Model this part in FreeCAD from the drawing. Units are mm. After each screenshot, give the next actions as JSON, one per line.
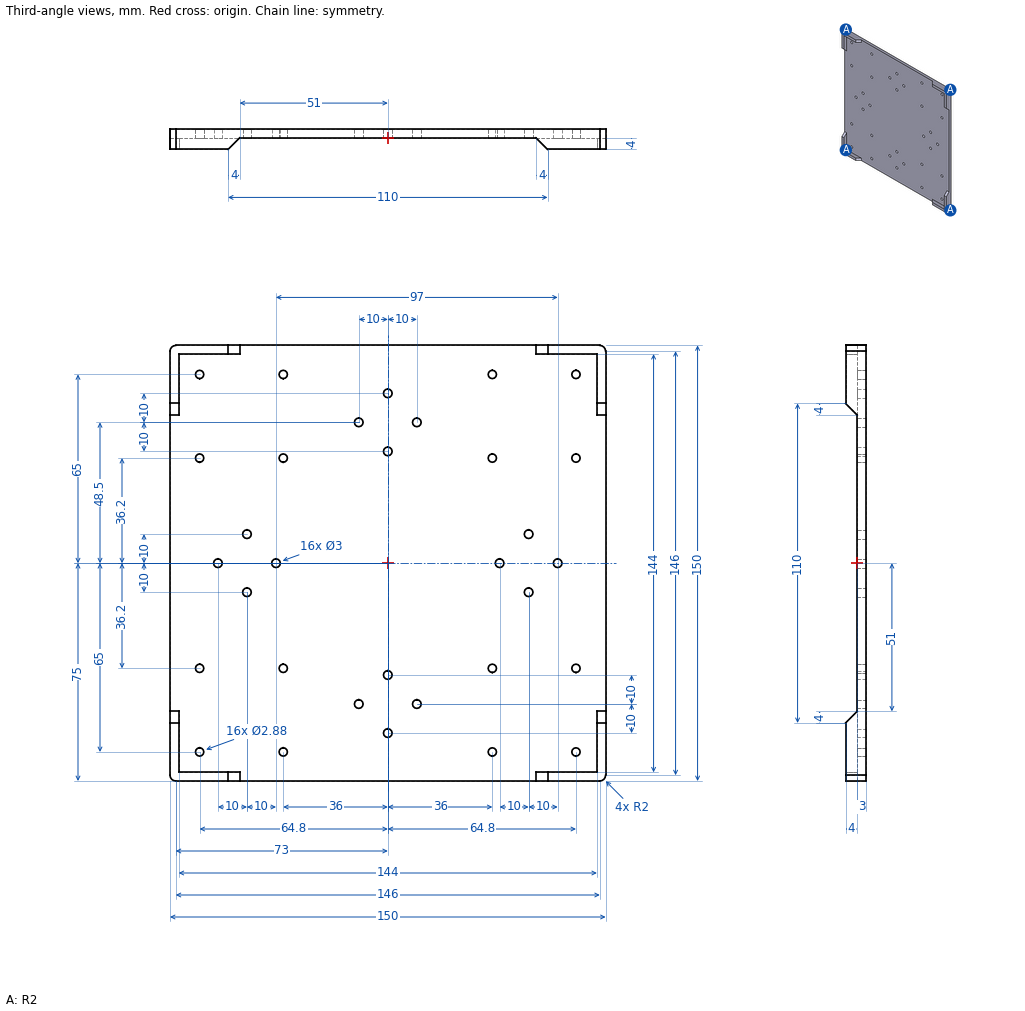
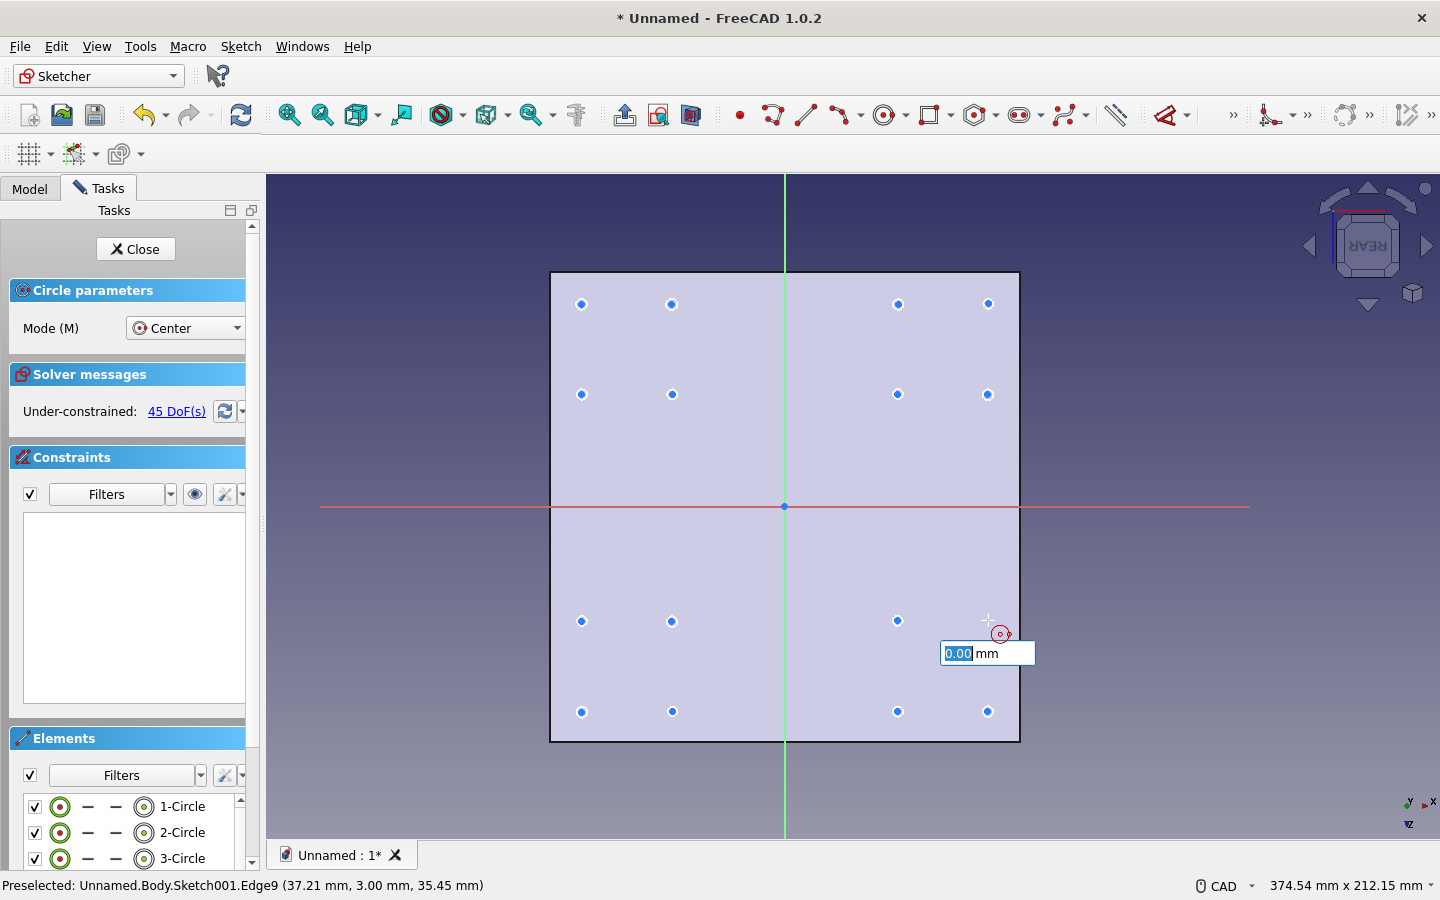
{"action": "scroll", "coordinate": [991, 617], "scroll_direction": "up", "scroll_amount": 7}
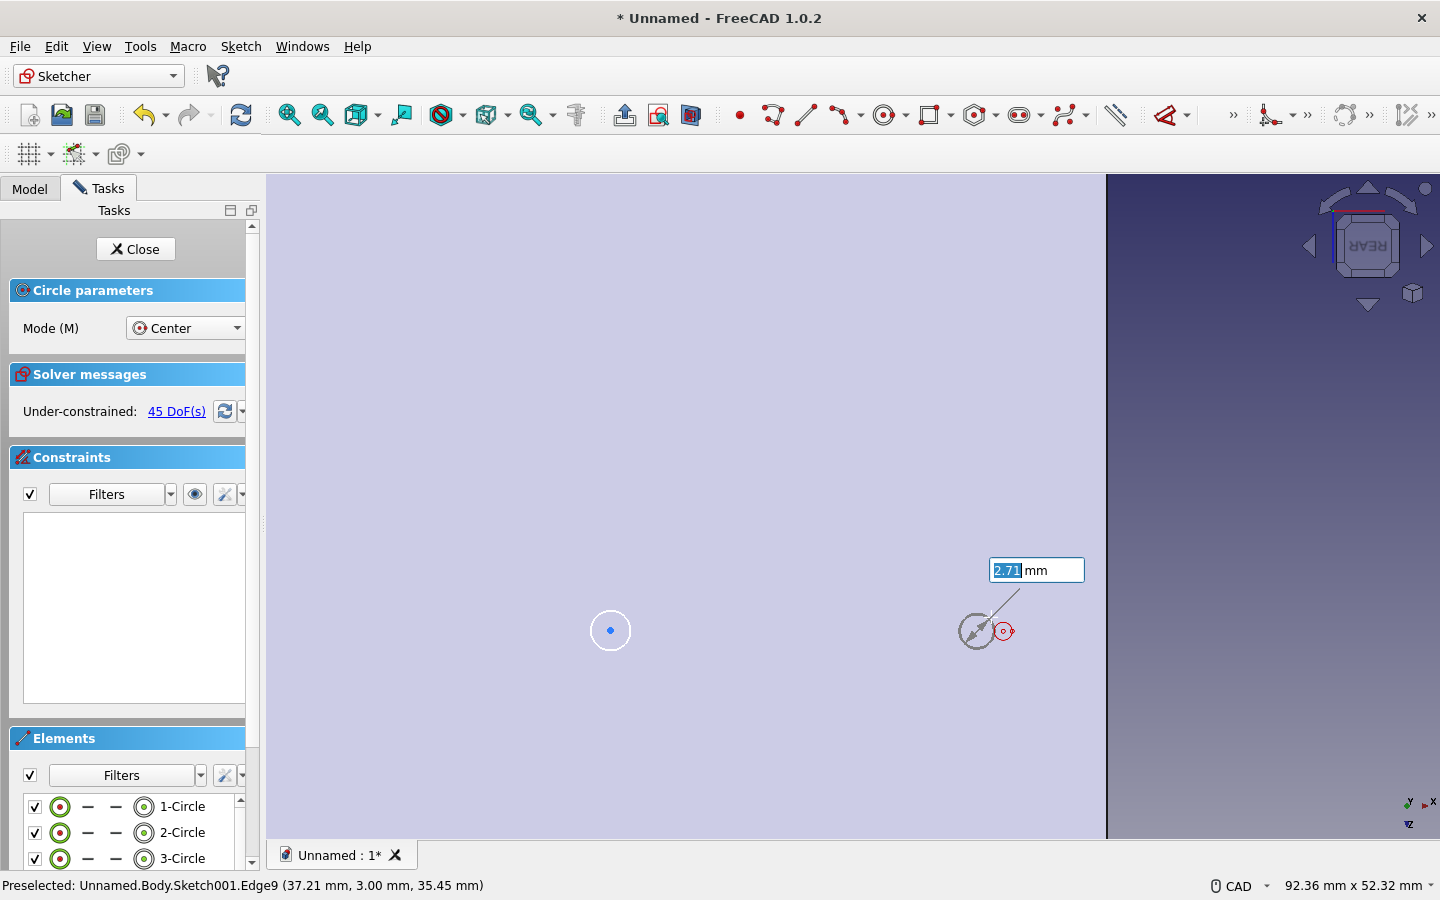
{"action": "left_click", "coordinate": [990, 616]}
{"action": "key", "text": "Escape"}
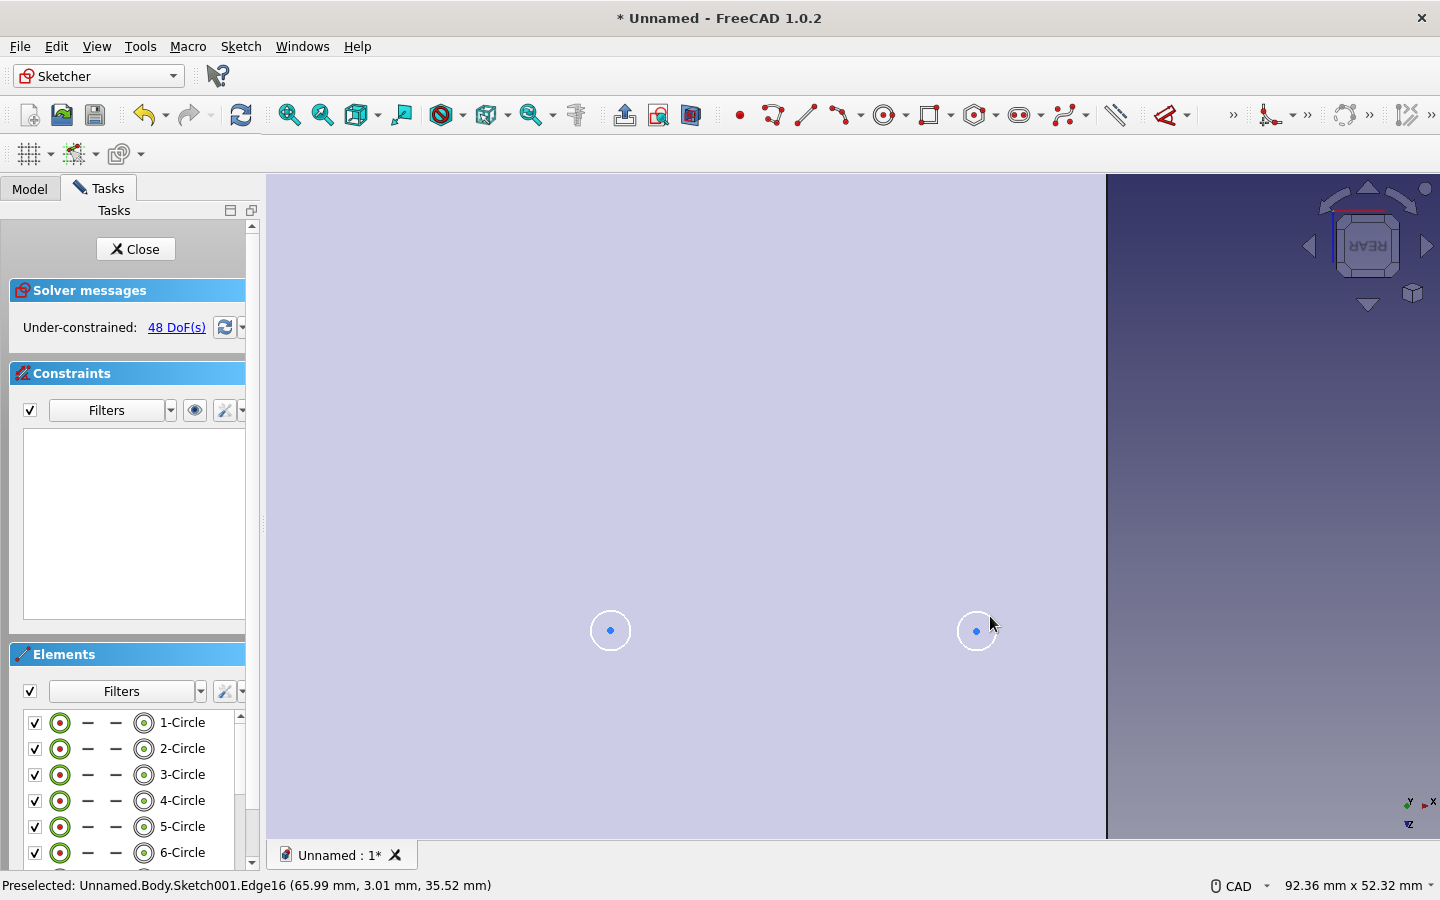
{"action": "scroll", "coordinate": [991, 617], "scroll_direction": "down", "scroll_amount": 7}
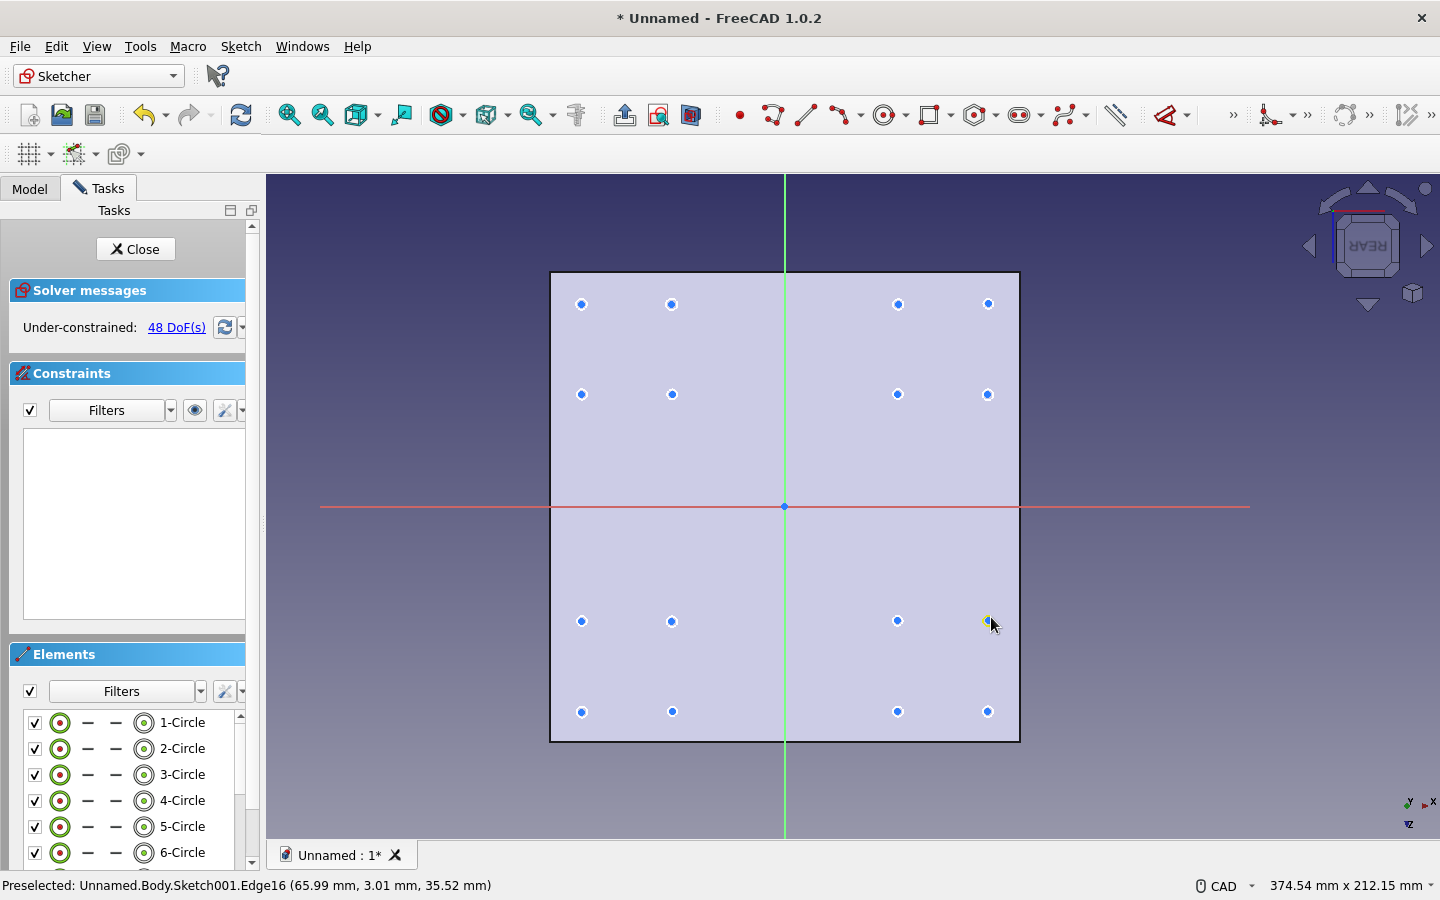
{"action": "scroll", "coordinate": [585, 301], "scroll_direction": "up", "scroll_amount": 5}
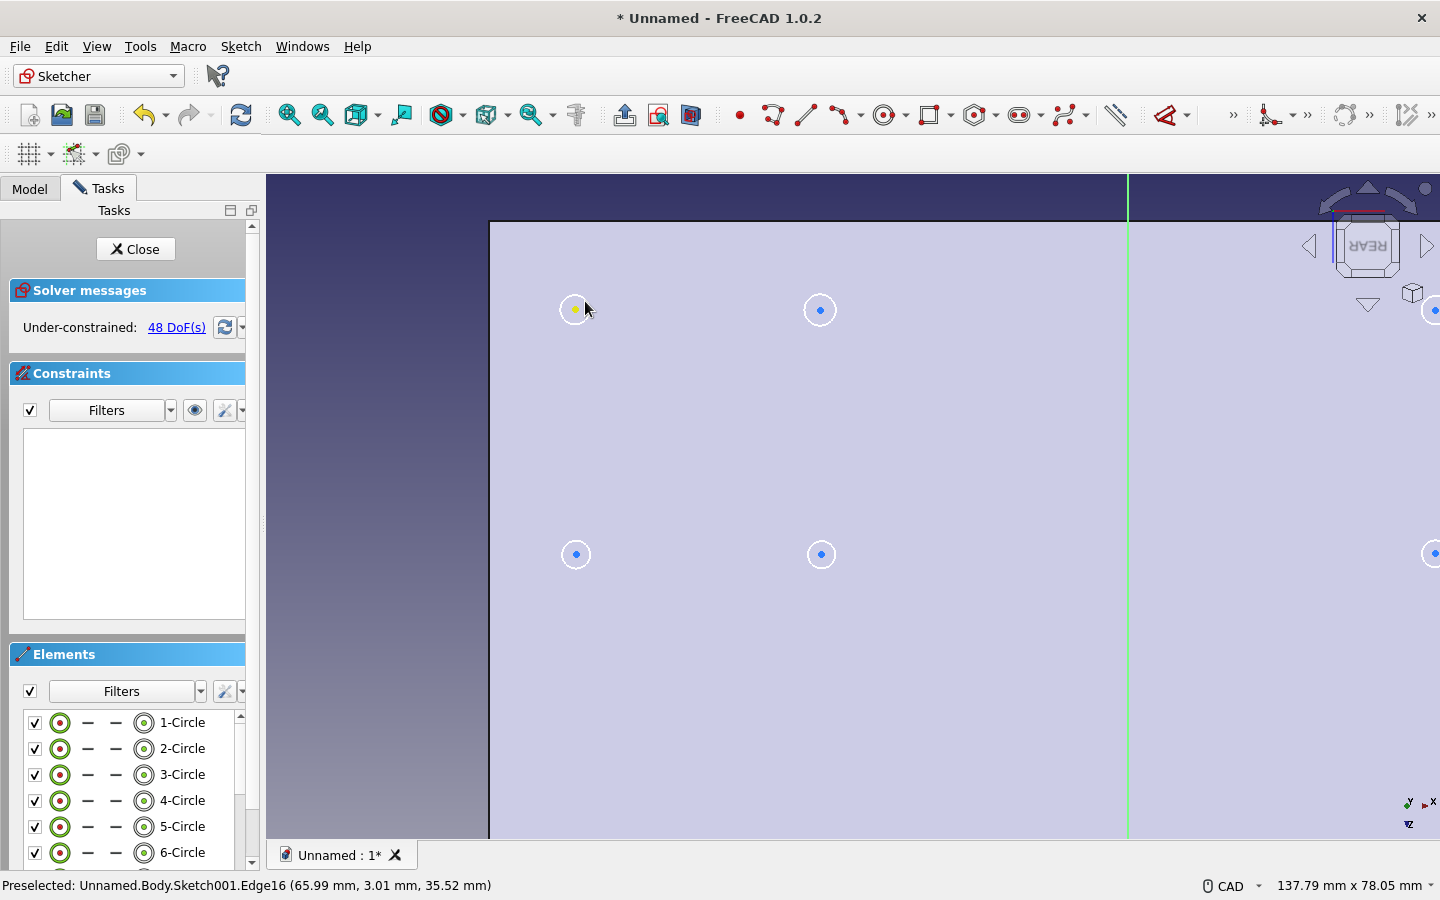
{"action": "left_click", "coordinate": [585, 299]}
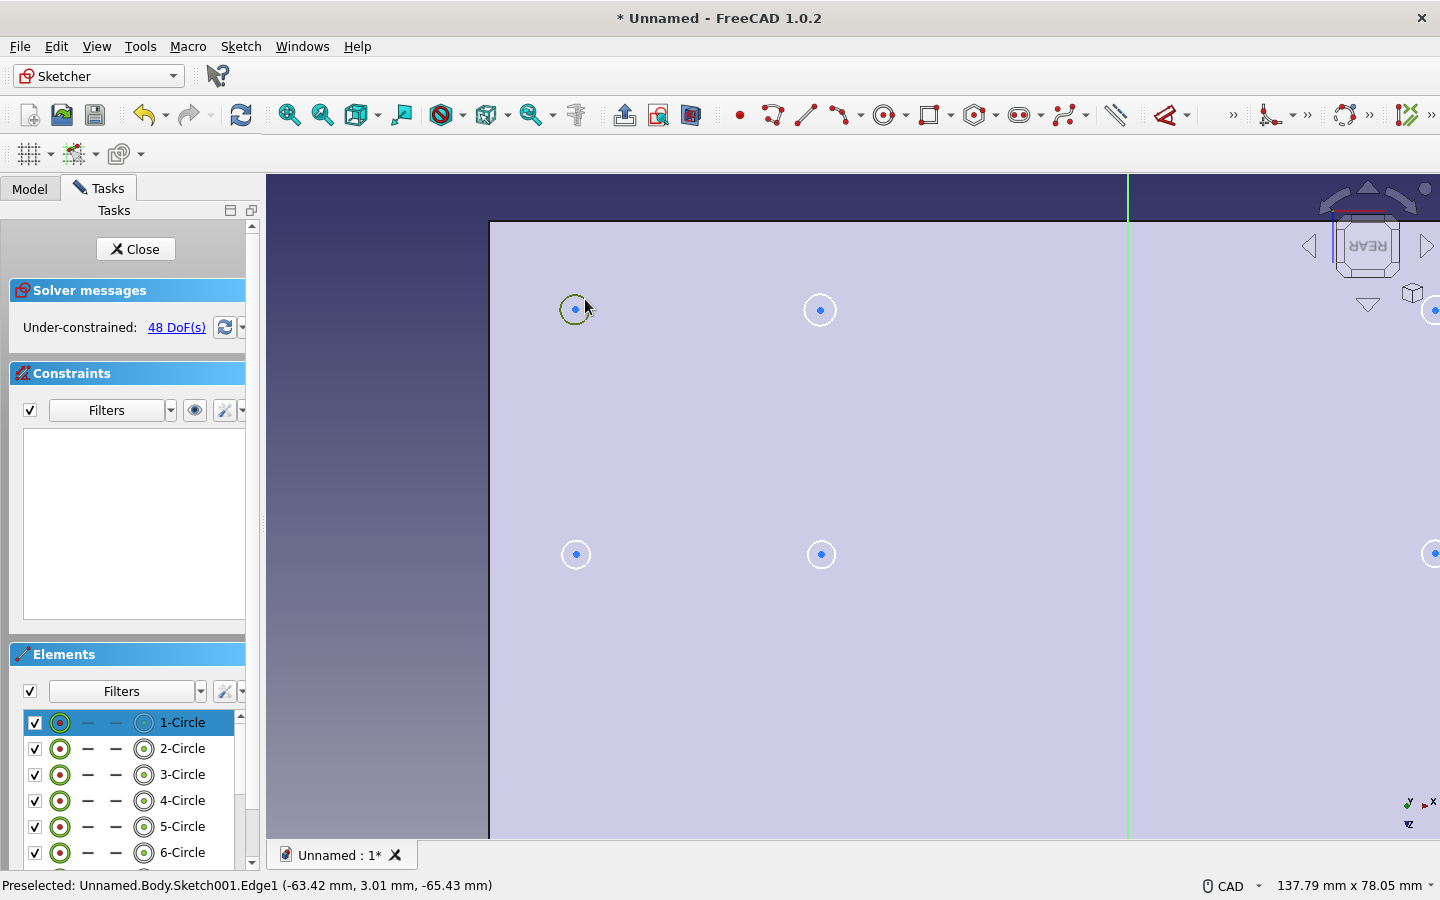
{"action": "left_click", "coordinate": [831, 299]}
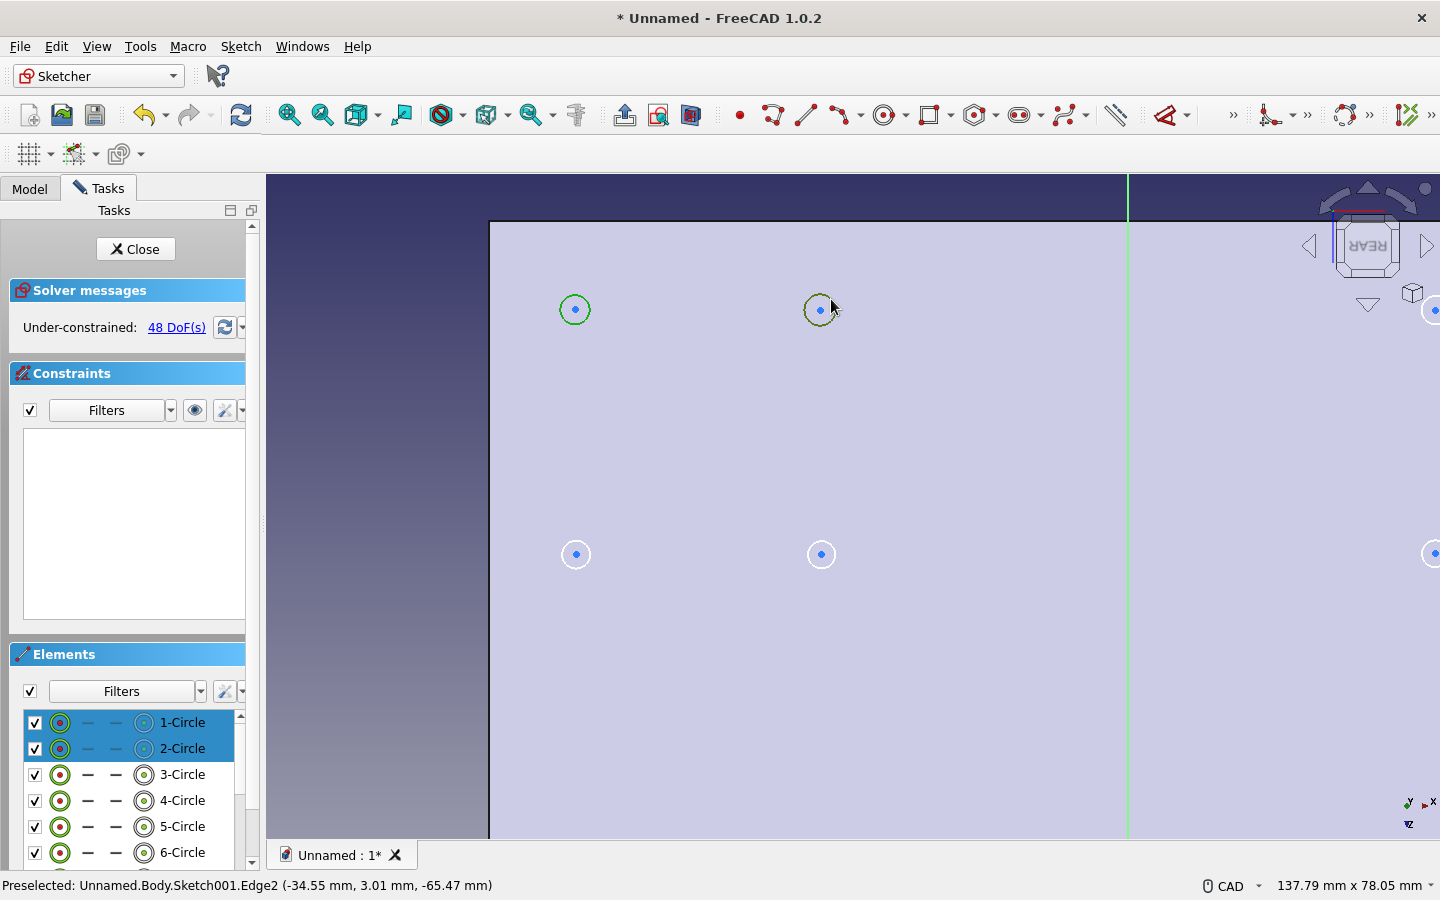
{"action": "left_click", "coordinate": [586, 545]}